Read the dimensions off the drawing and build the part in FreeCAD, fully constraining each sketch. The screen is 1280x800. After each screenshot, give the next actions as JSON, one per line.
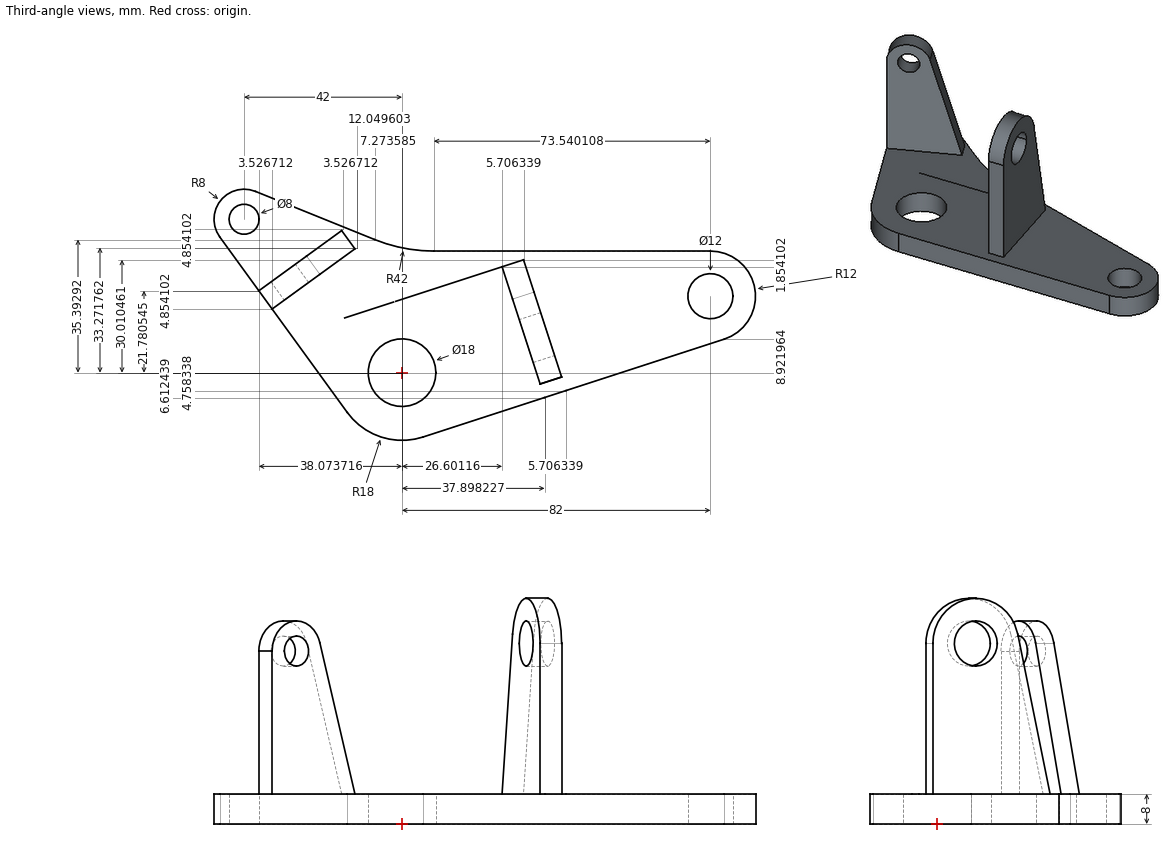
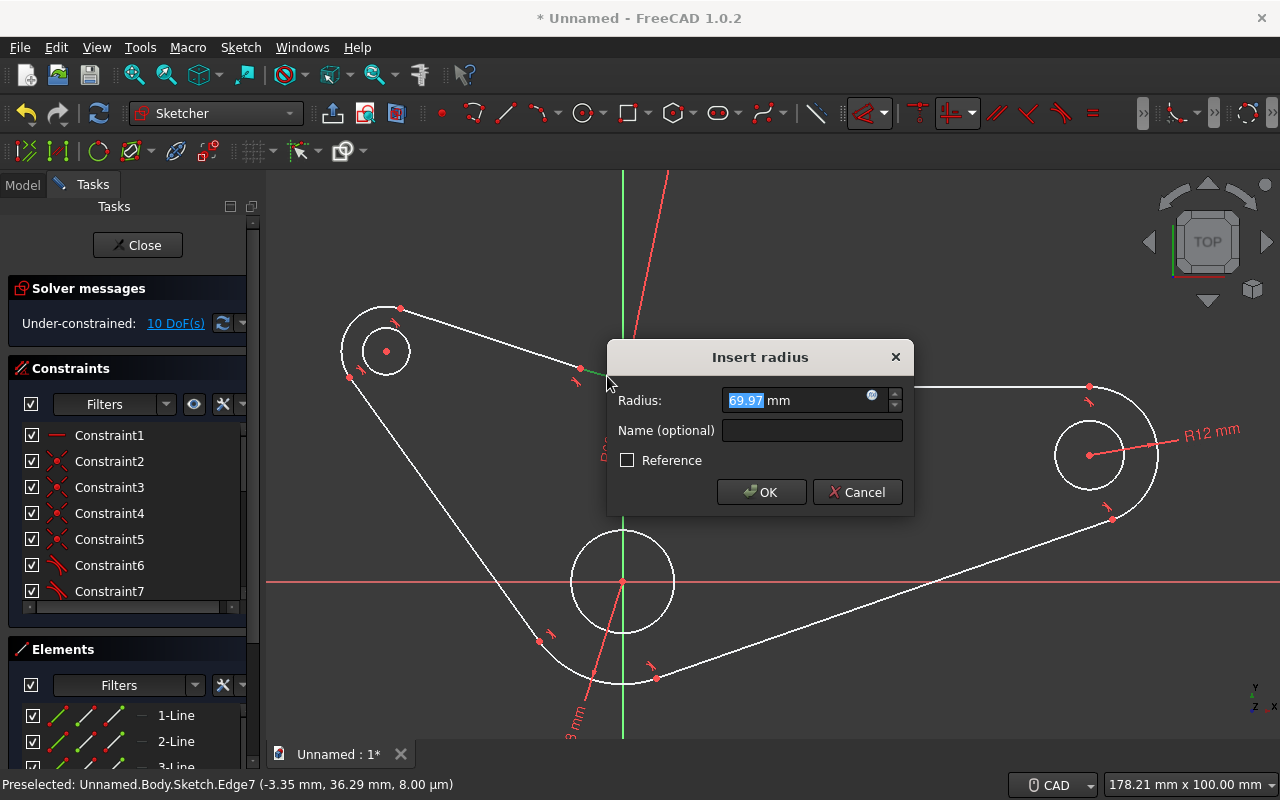
{"action": "type", "text": "42"}
{"action": "key", "text": "Return"}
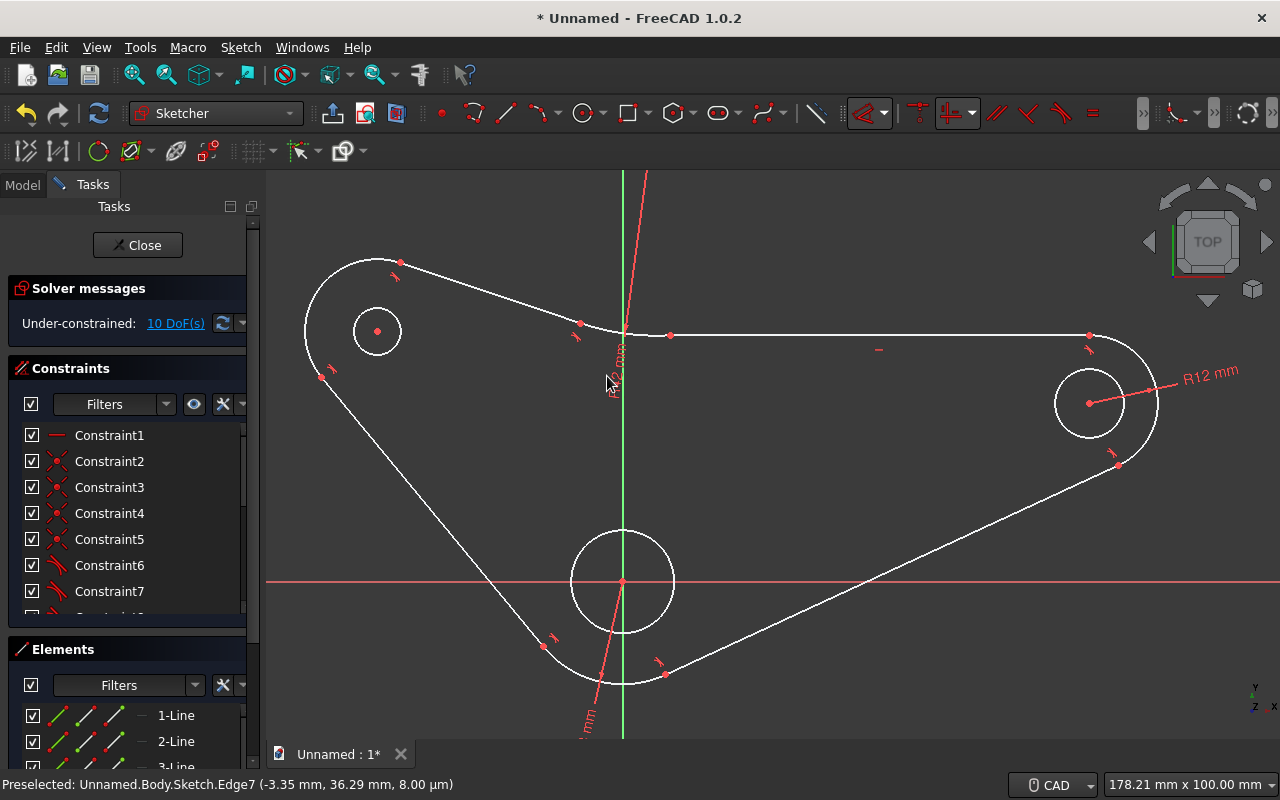
{"action": "left_click", "coordinate": [346, 266]}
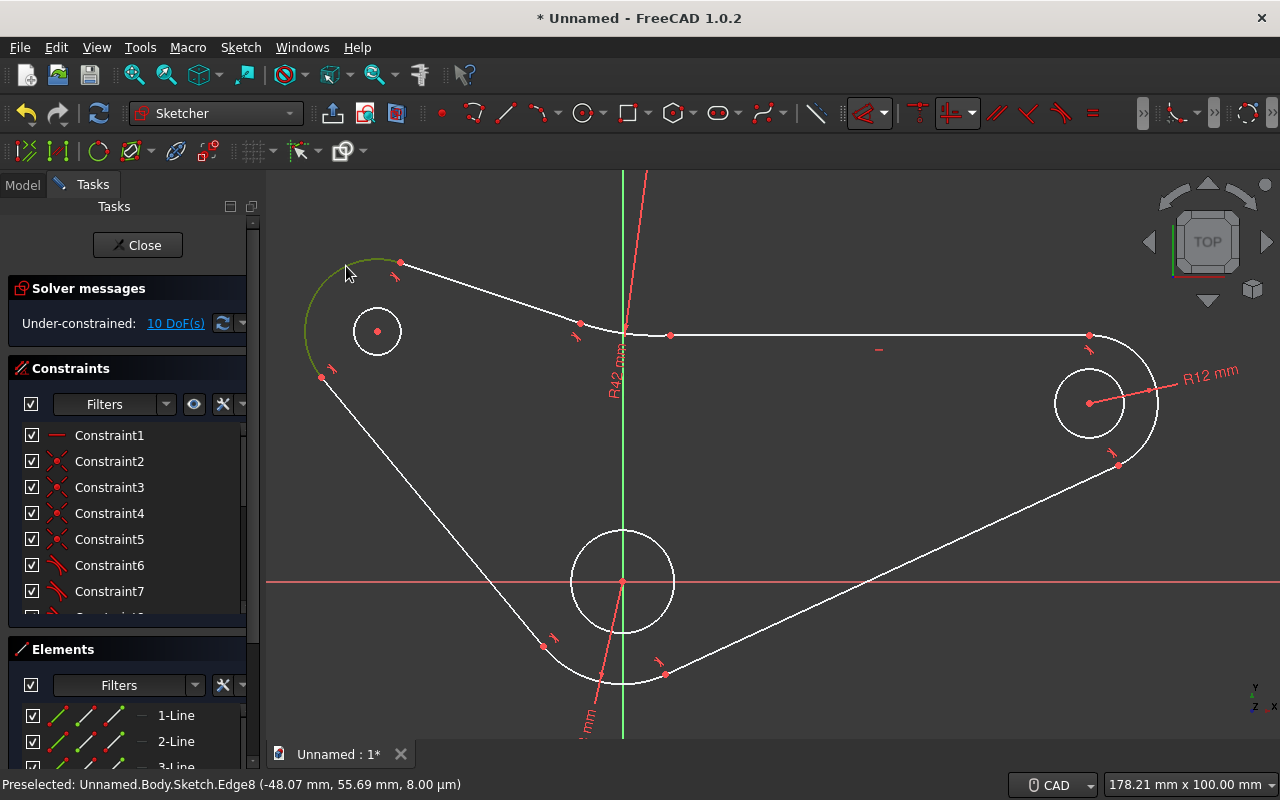
{"action": "key", "text": "k r"}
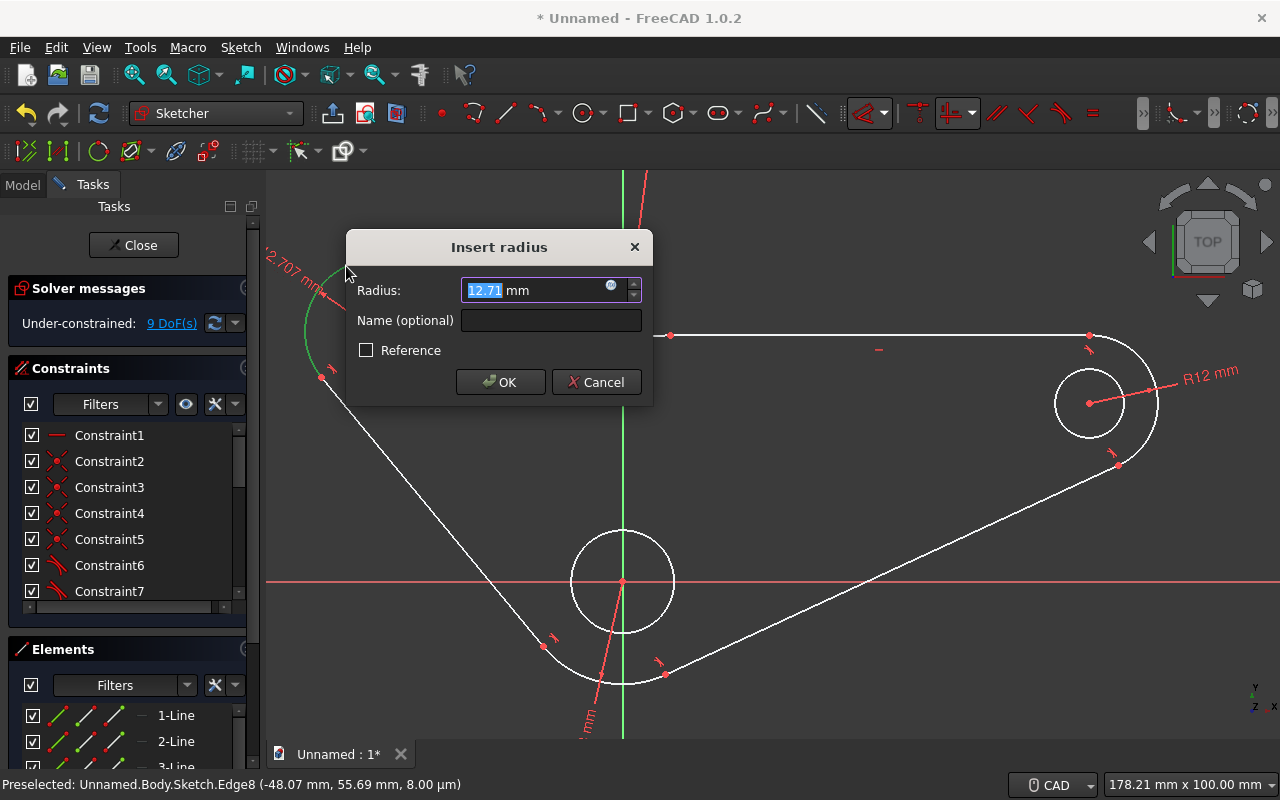
{"action": "type", "text": "8"}
{"action": "key", "text": "Return"}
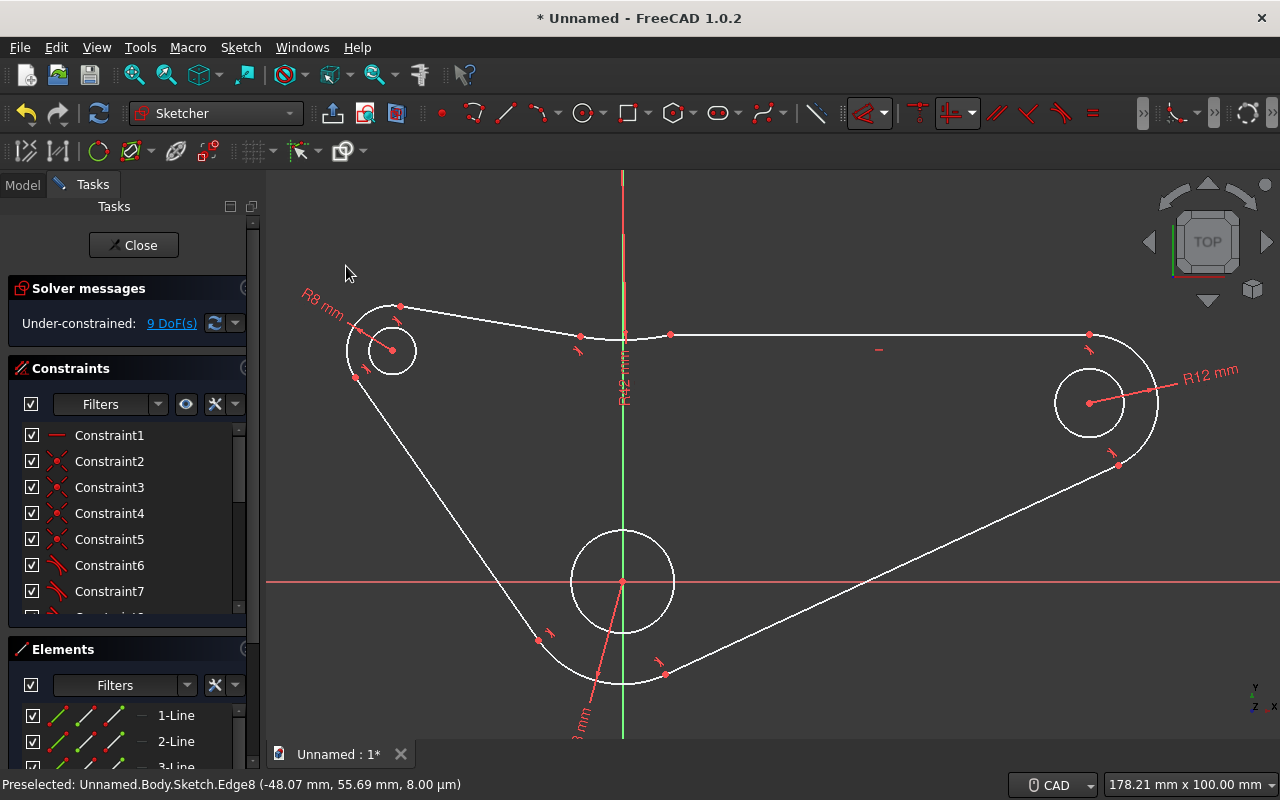
{"action": "left_click", "coordinate": [659, 545]}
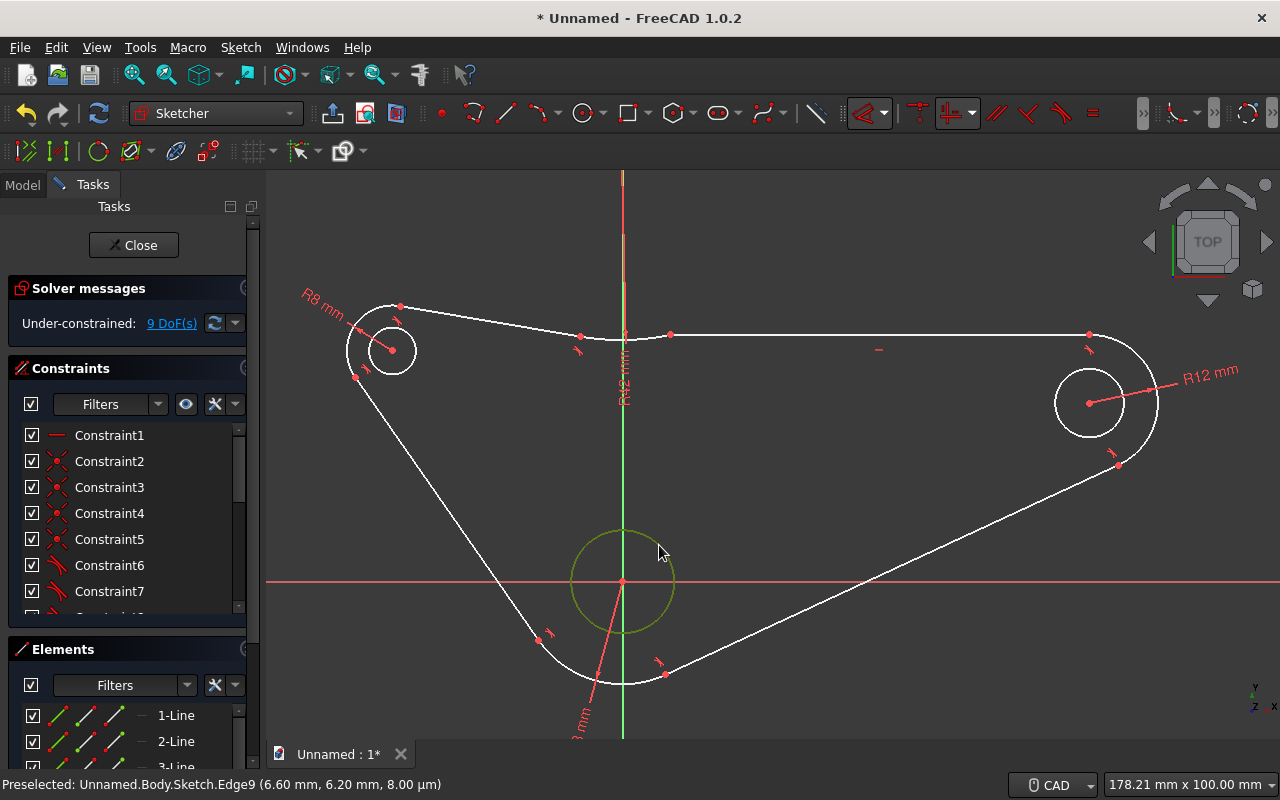
{"action": "key", "text": "k o"}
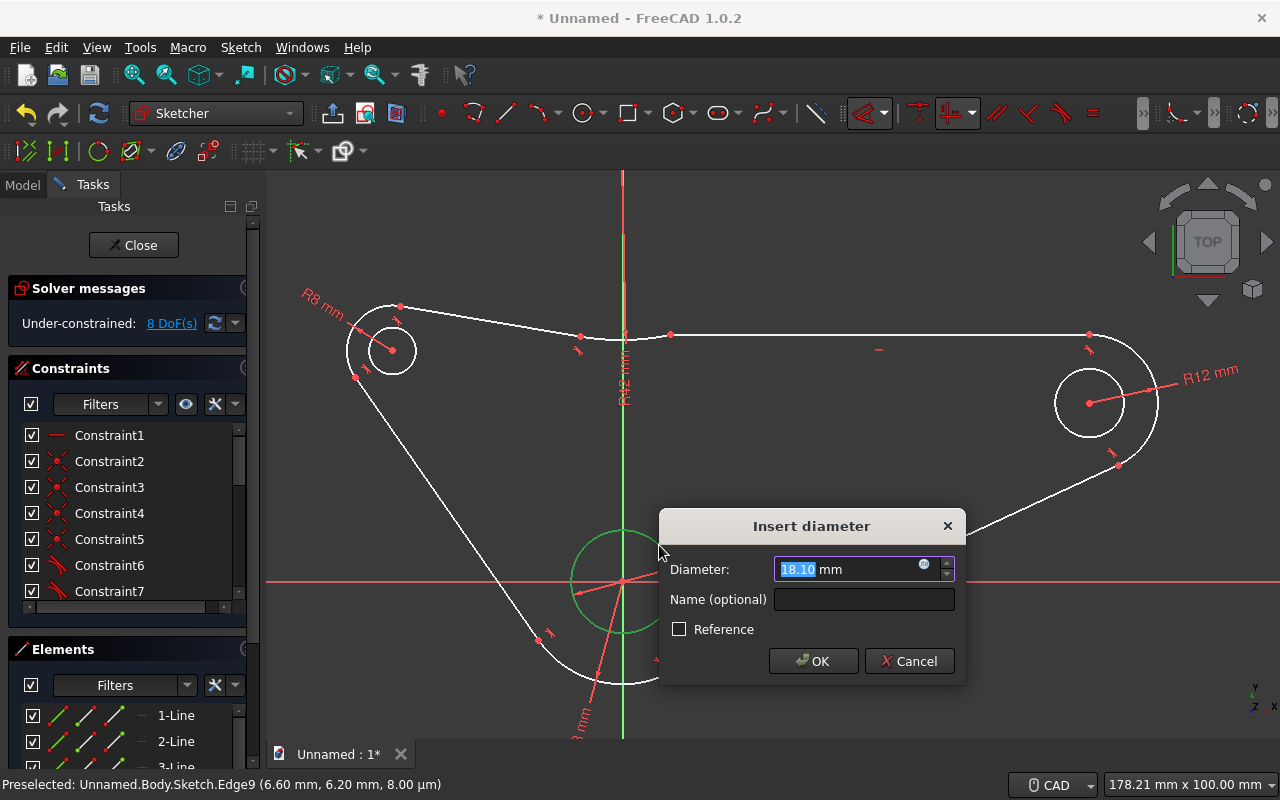
{"action": "type", "text": "18"}
{"action": "key", "text": "Return"}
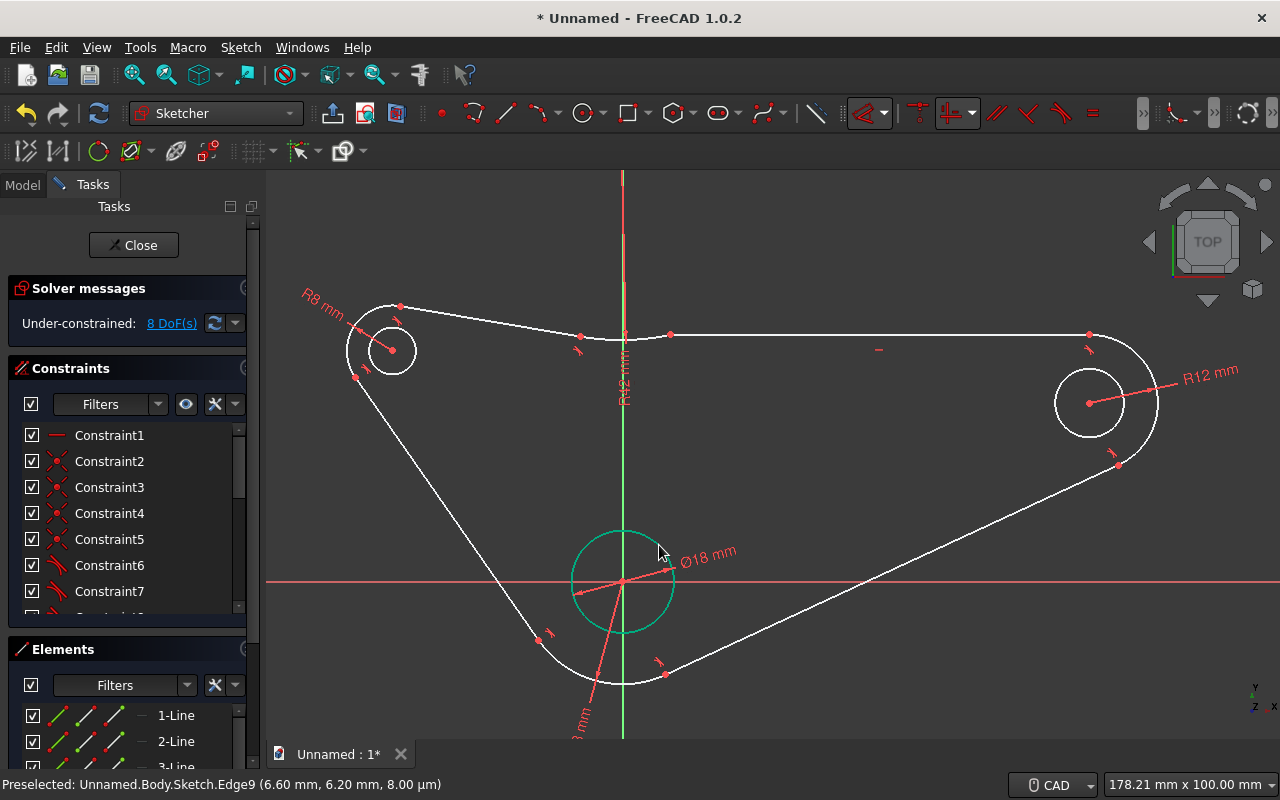
{"action": "left_click", "coordinate": [409, 334]}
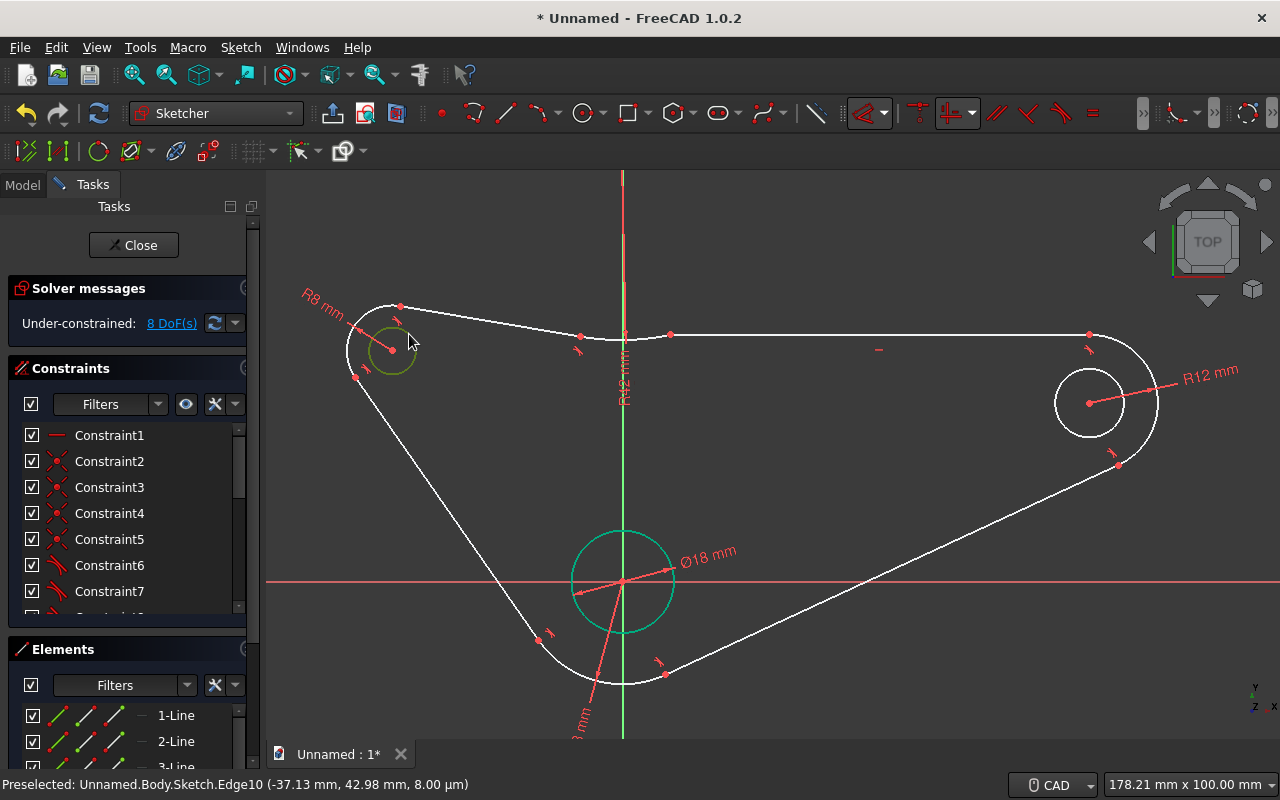
{"action": "key", "text": "k o"}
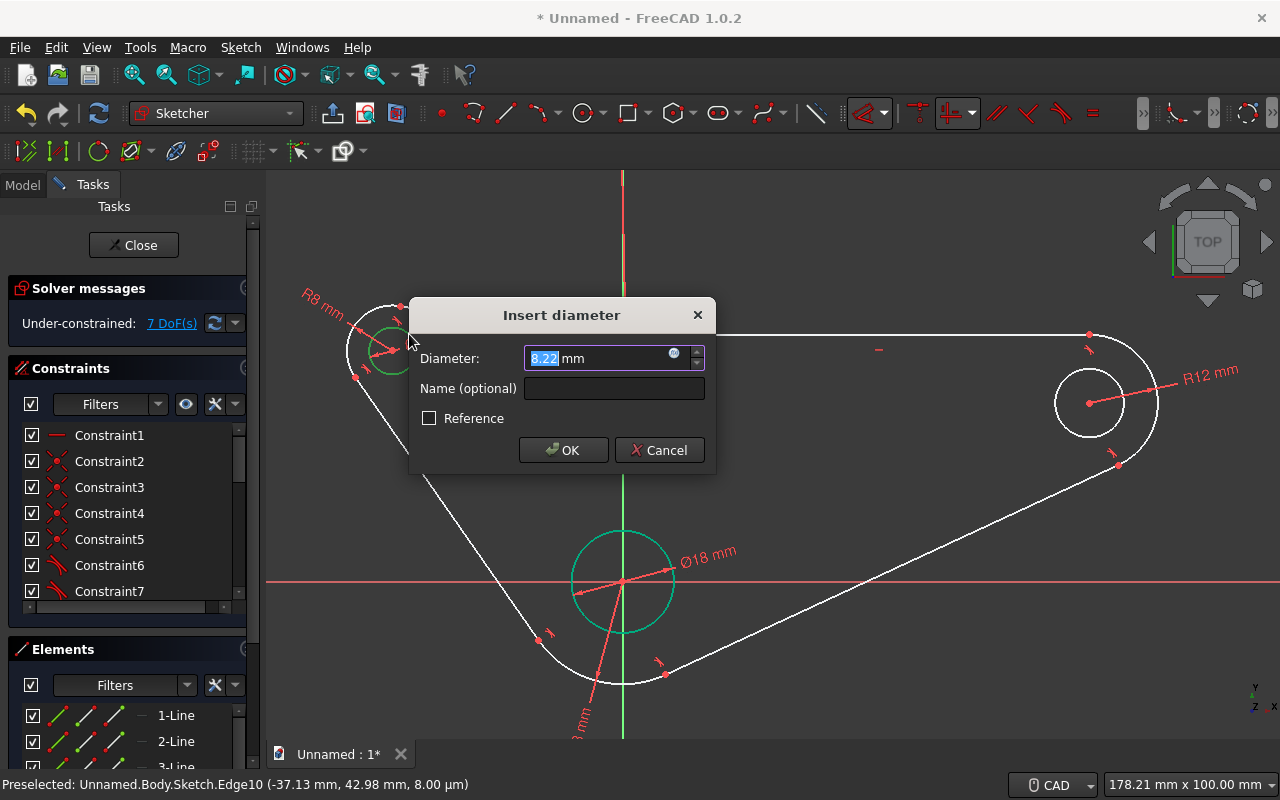
{"action": "type", "text": "8"}
{"action": "key", "text": "Return"}